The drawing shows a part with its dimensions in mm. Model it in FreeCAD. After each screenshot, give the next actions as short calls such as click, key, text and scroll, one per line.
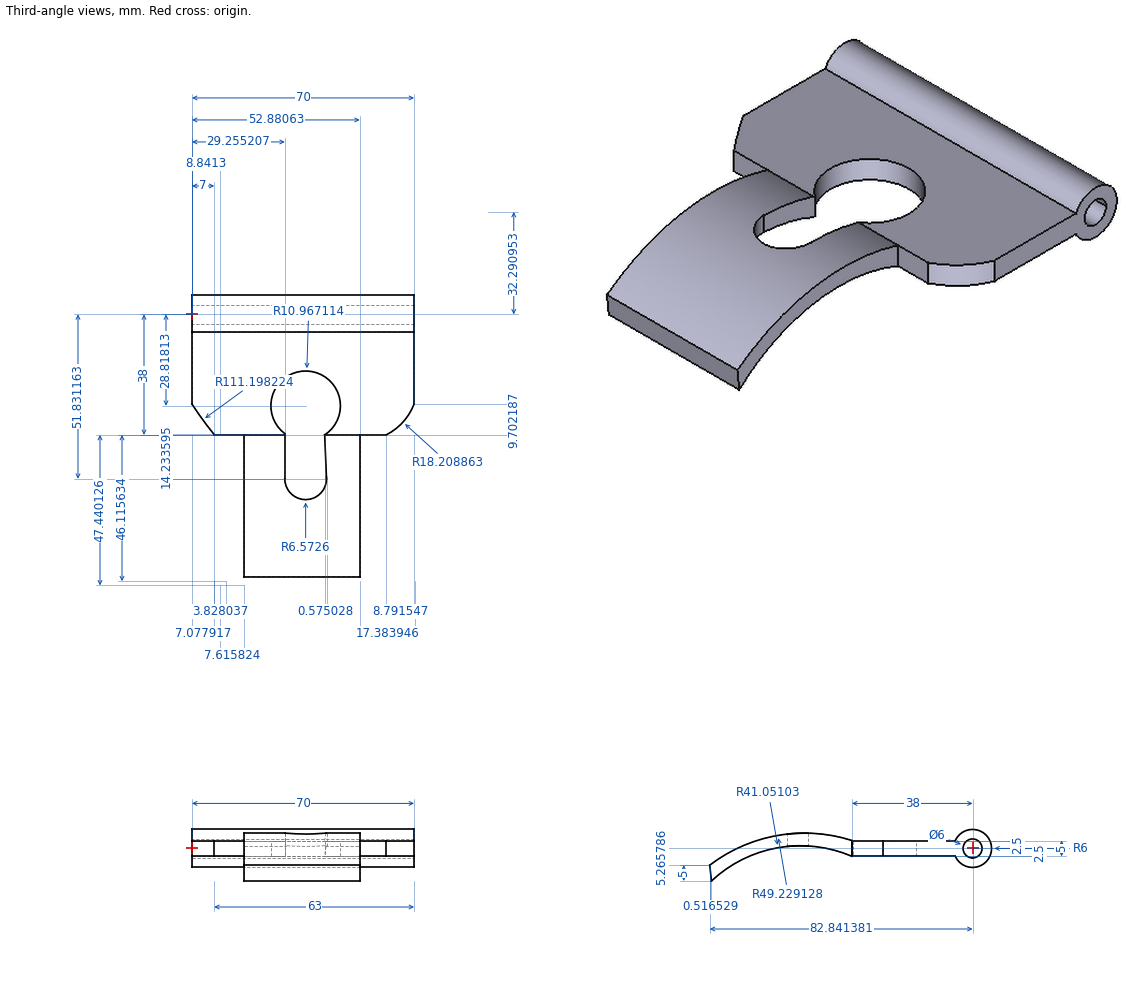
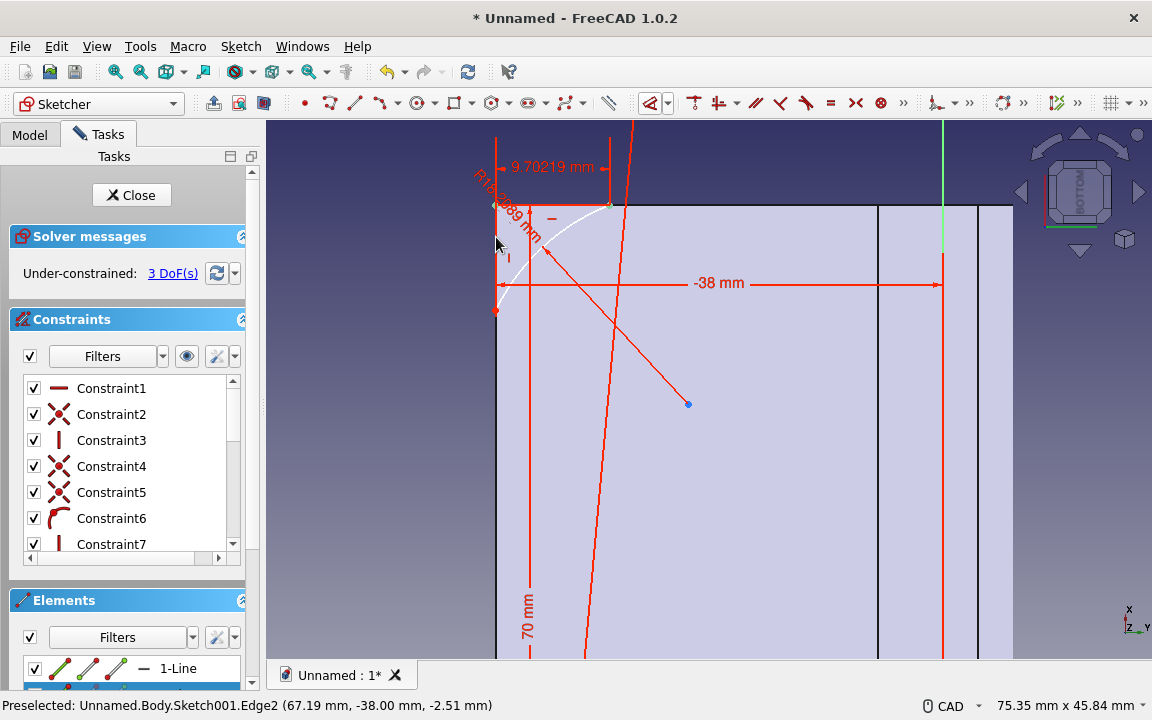
key(i)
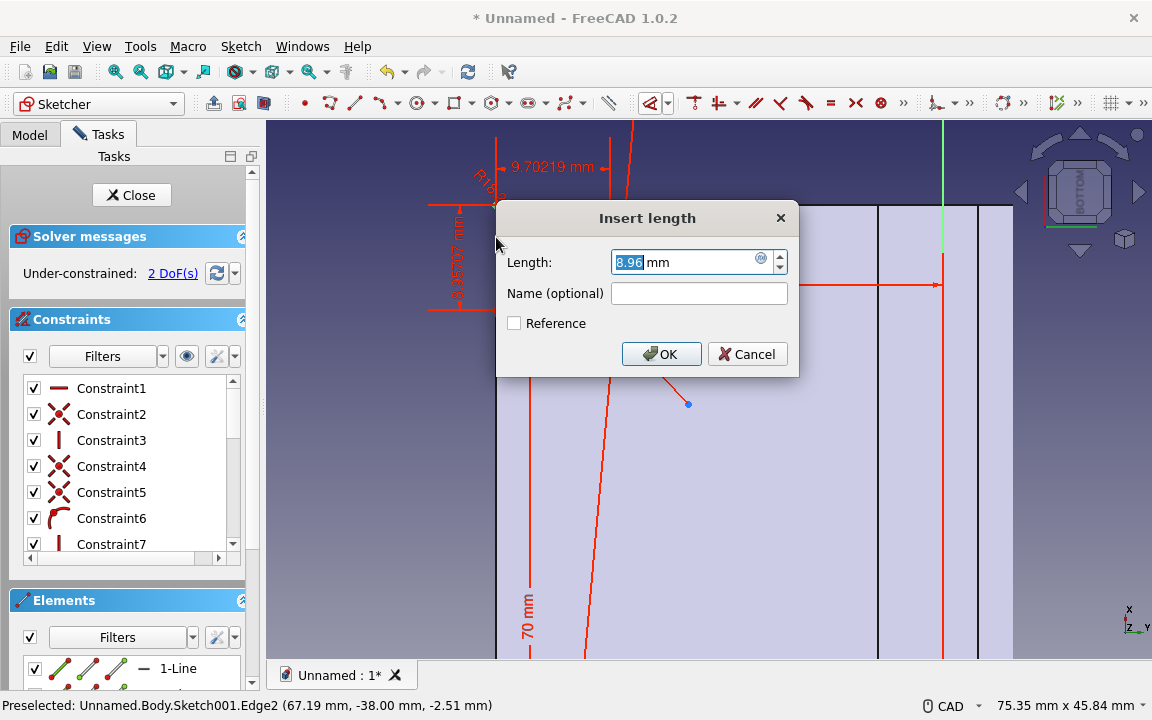
text(8.791547)
key(Return)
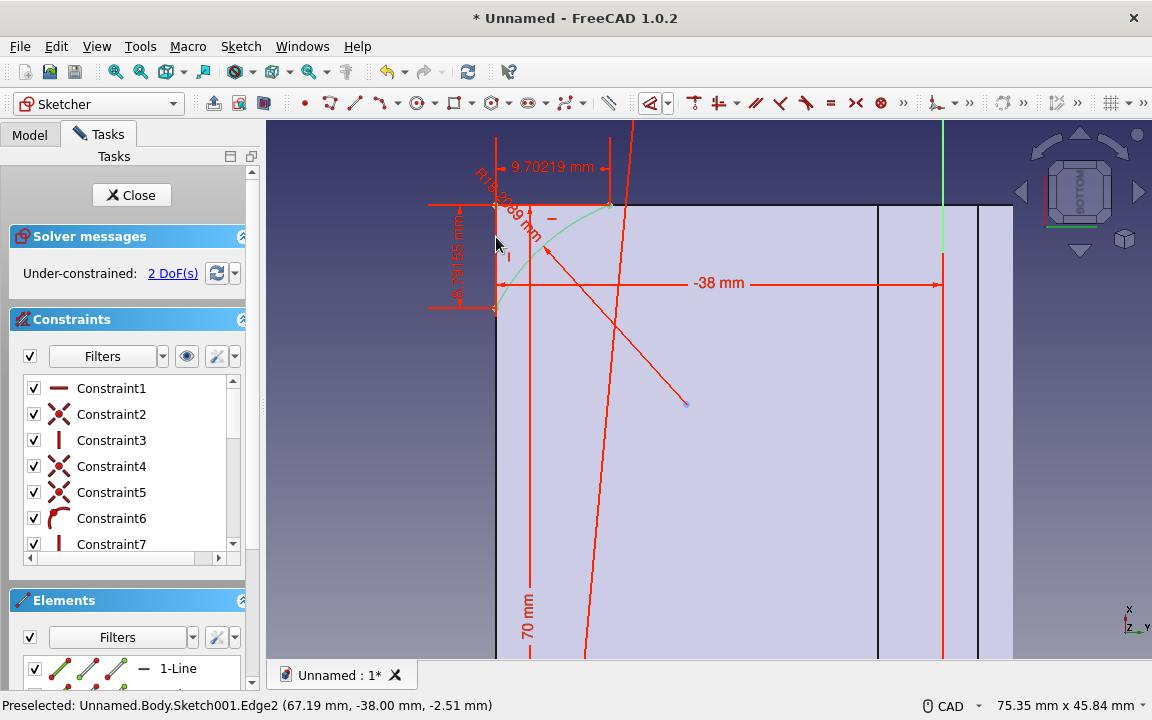
scroll(576, 204, down, 4)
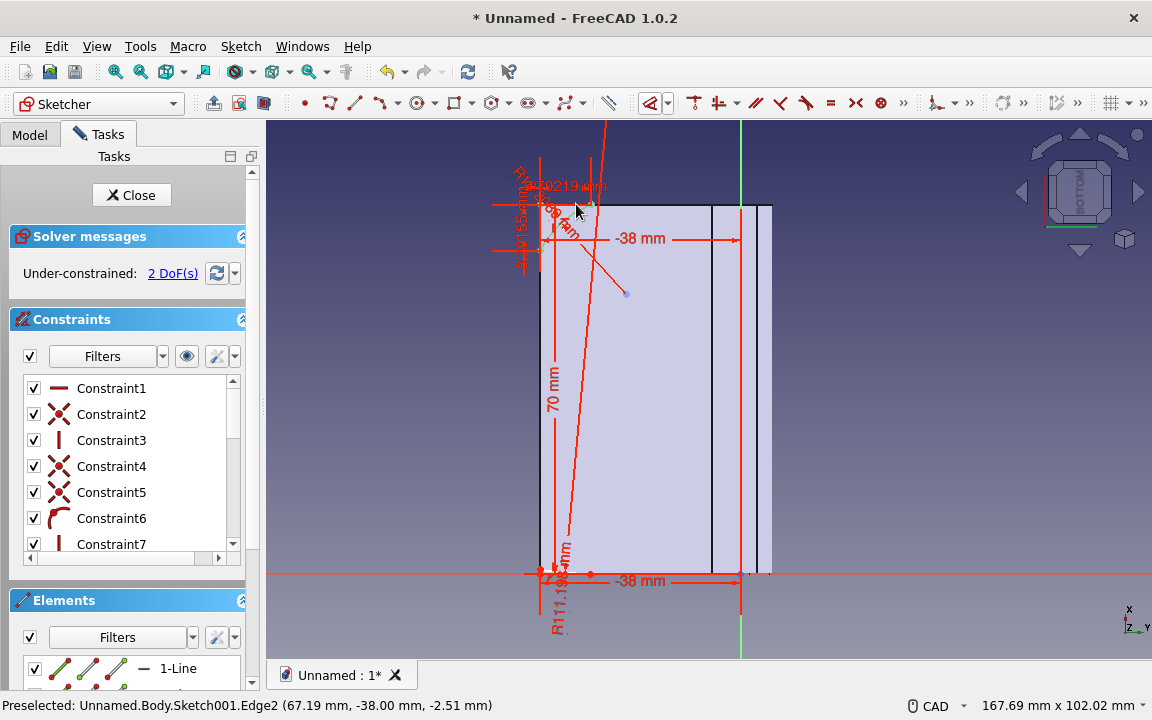
scroll(540, 572, up, 10)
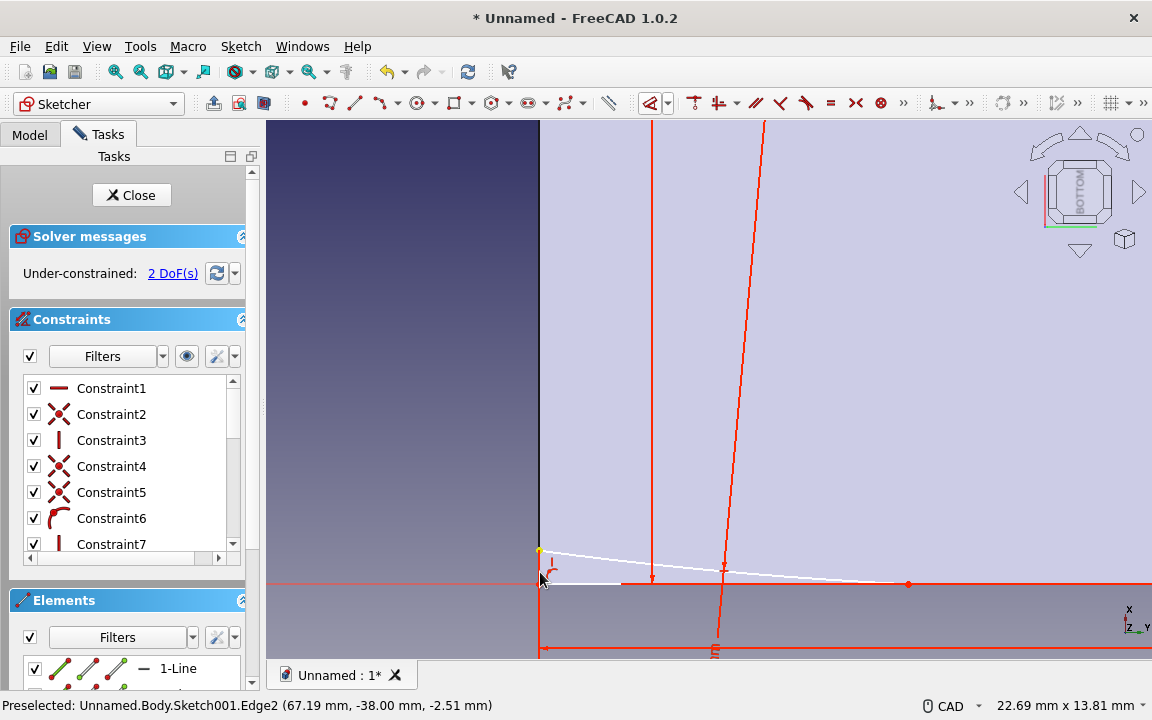
click(539, 567)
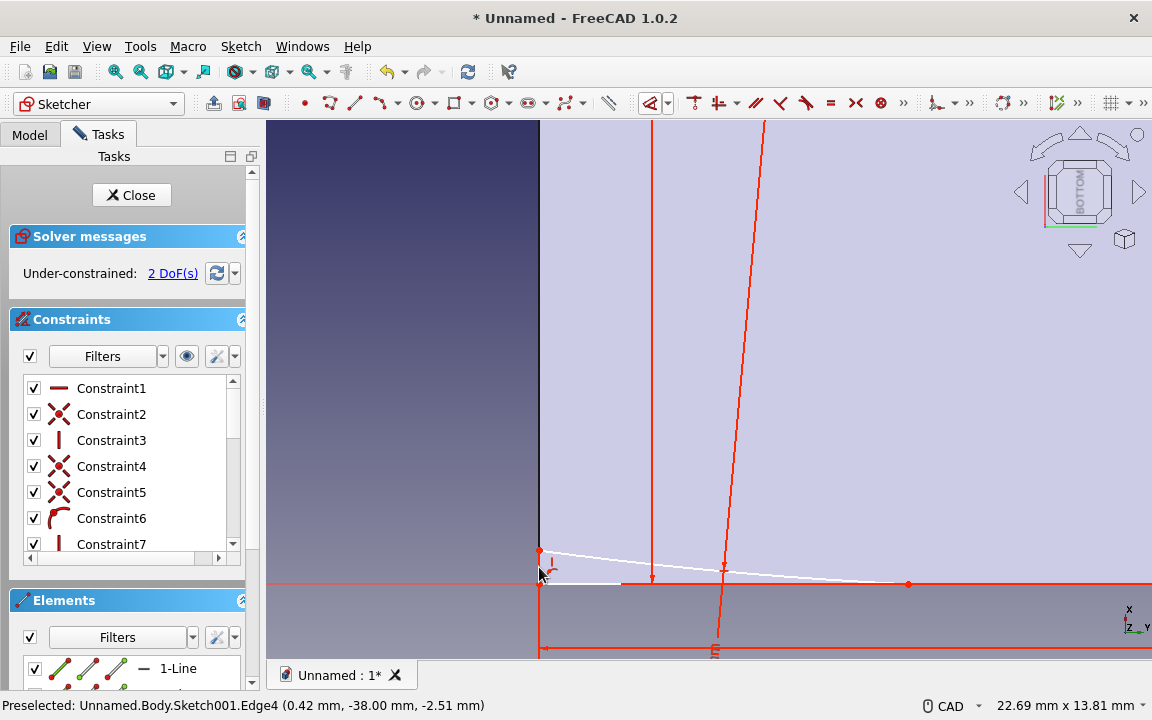
click(668, 104)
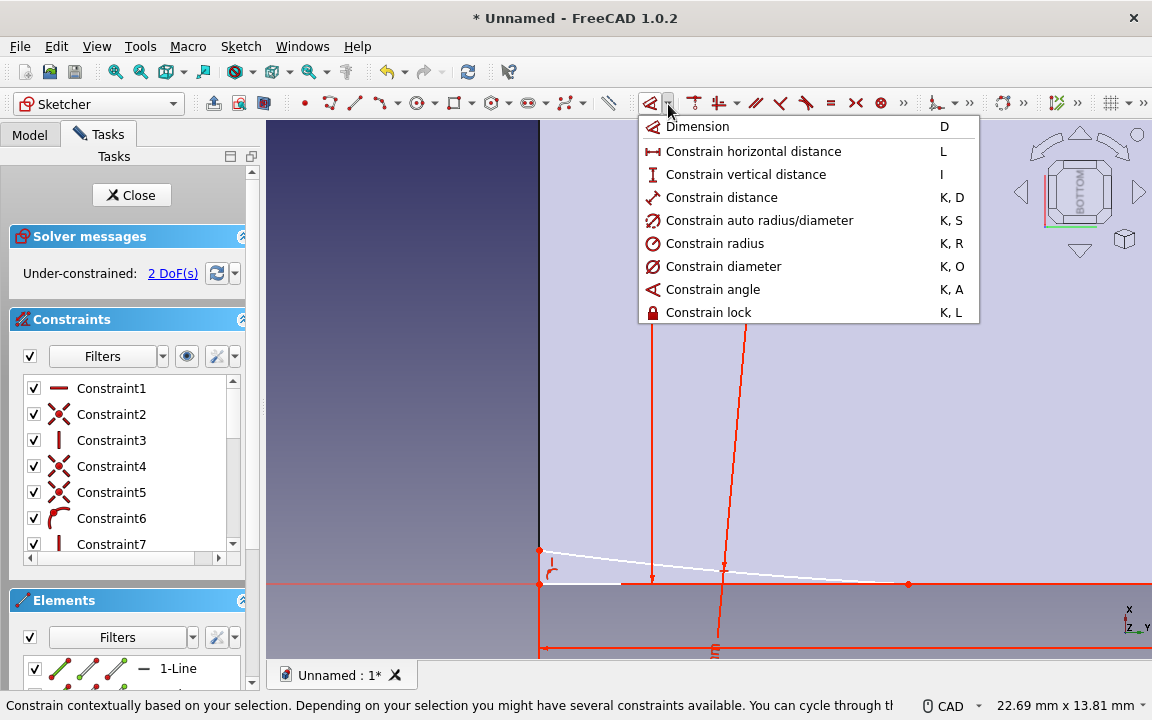
click(809, 174)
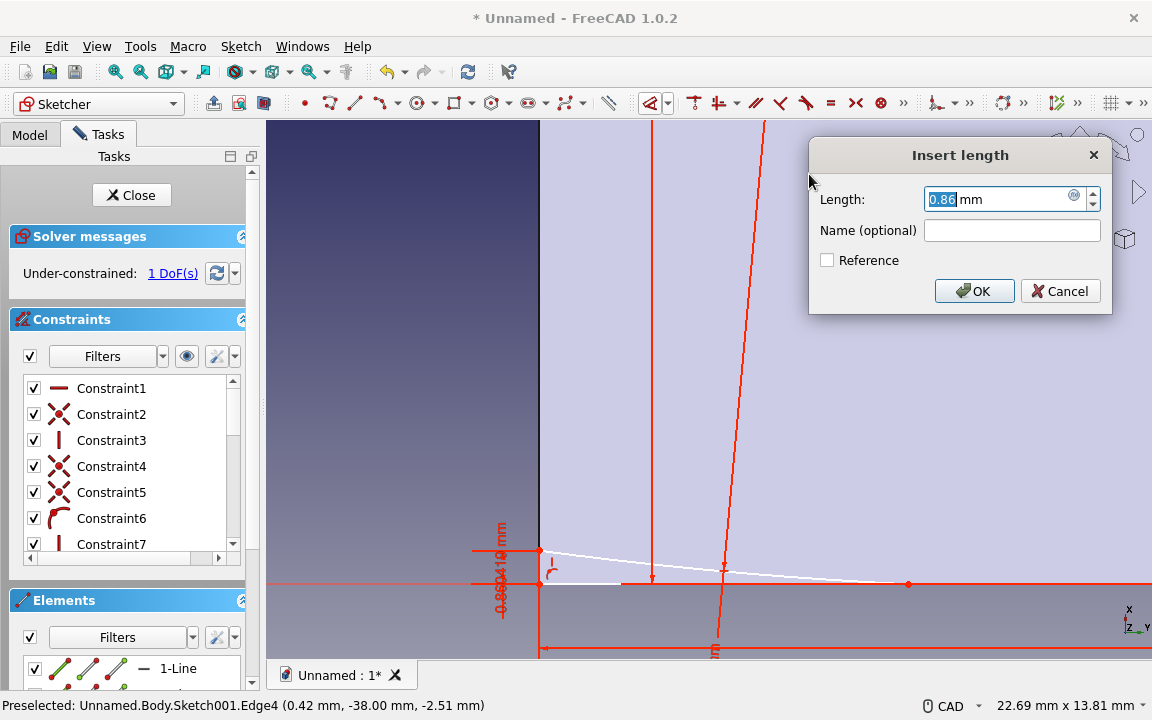
text(7.077917)
key(Return)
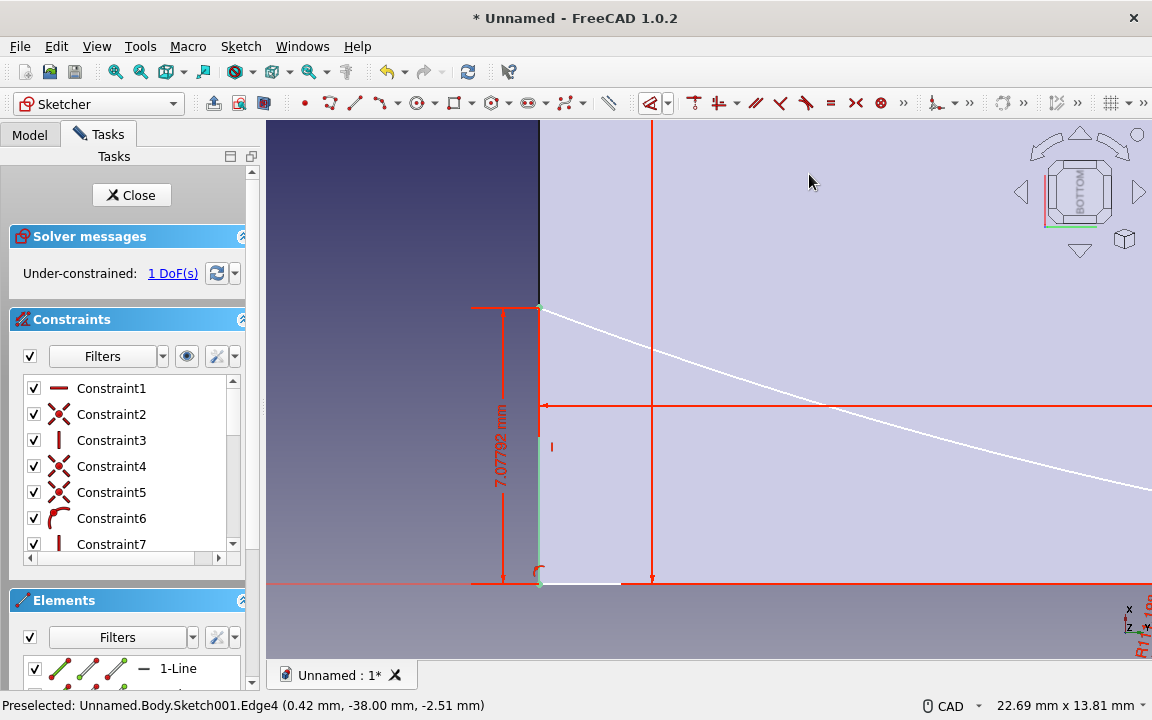
scroll(540, 573, down, 10)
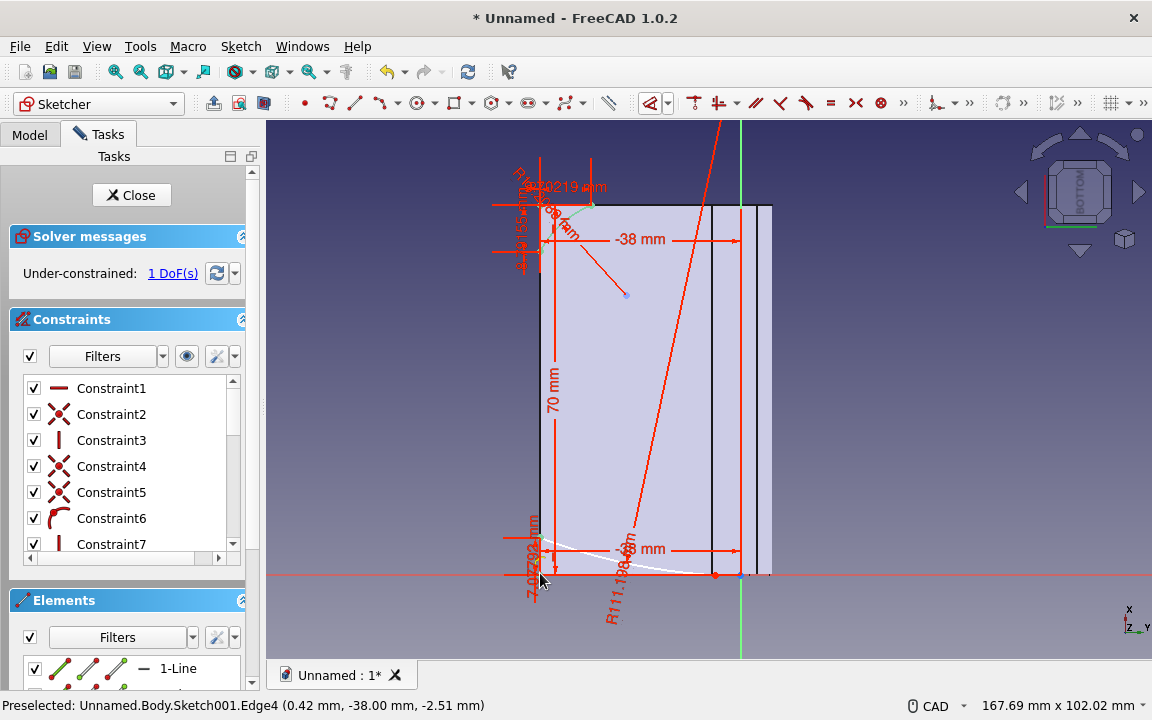
scroll(636, 520, down, 3)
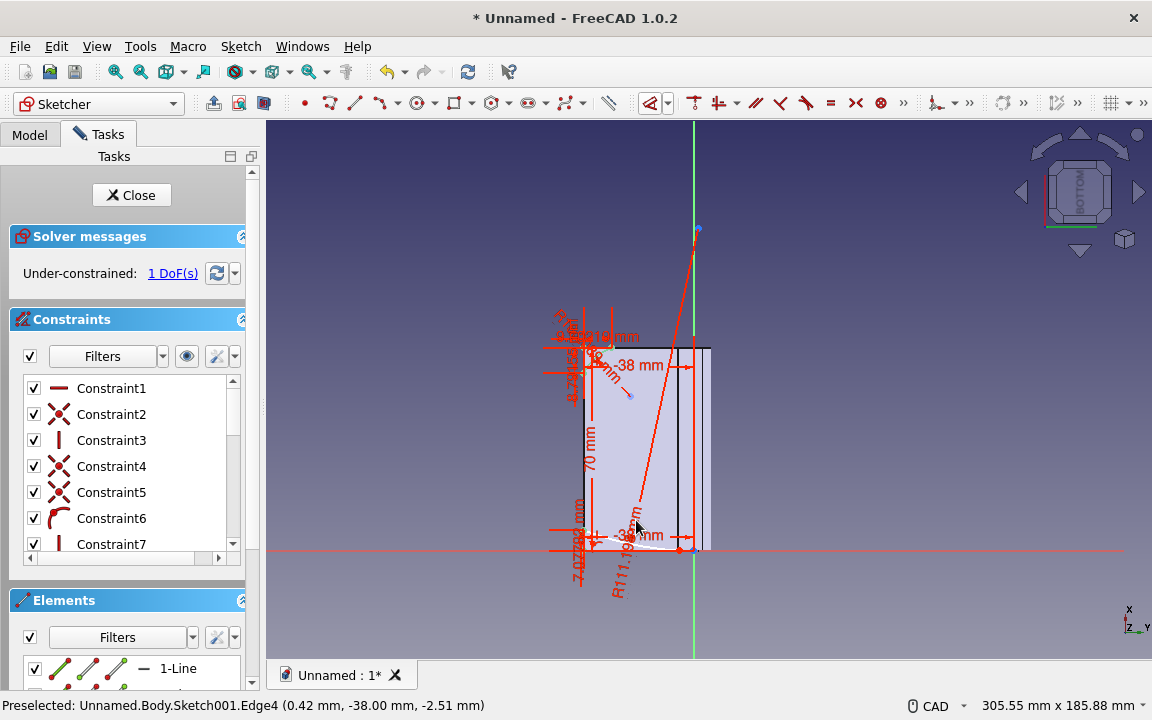
click(698, 229)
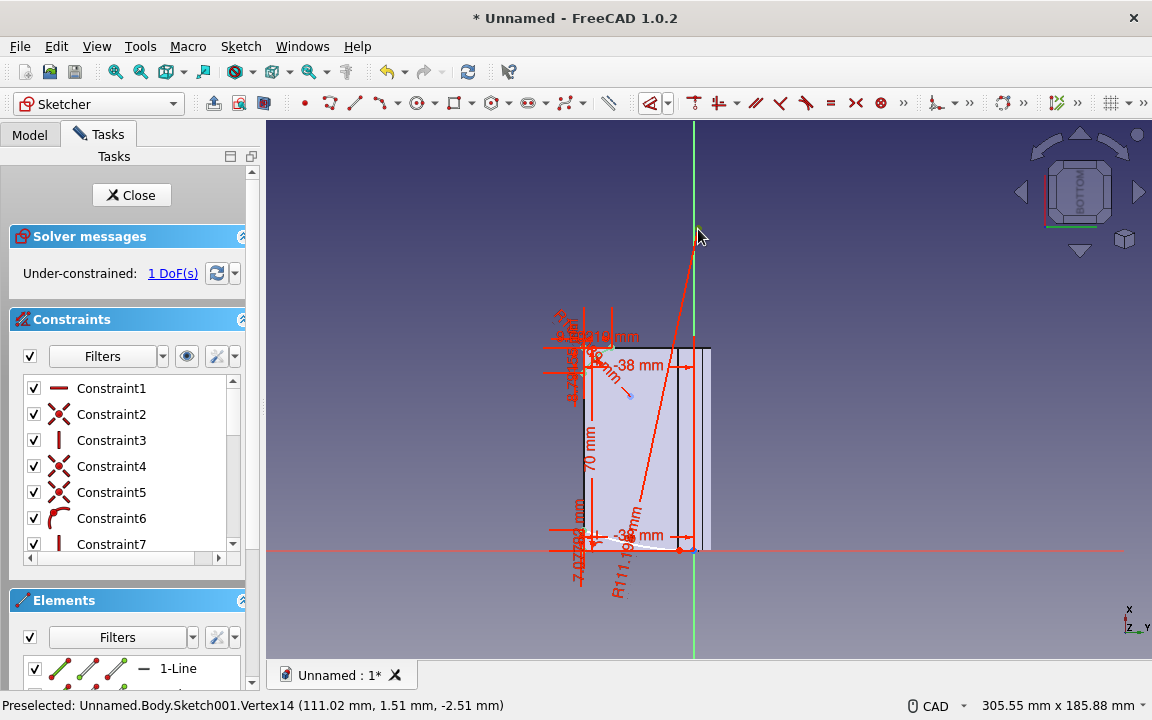
key(l)